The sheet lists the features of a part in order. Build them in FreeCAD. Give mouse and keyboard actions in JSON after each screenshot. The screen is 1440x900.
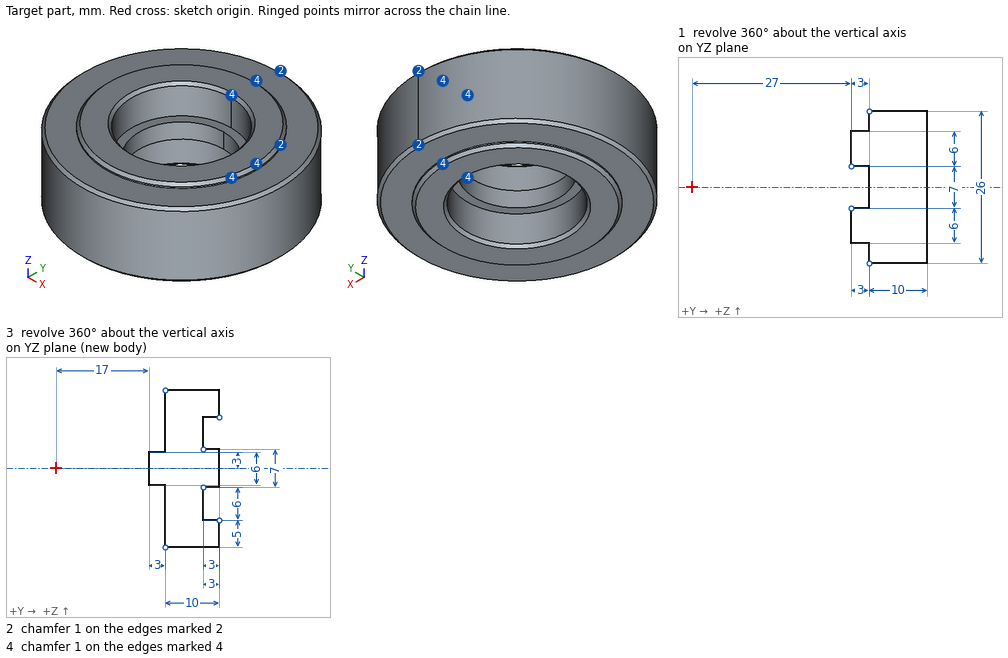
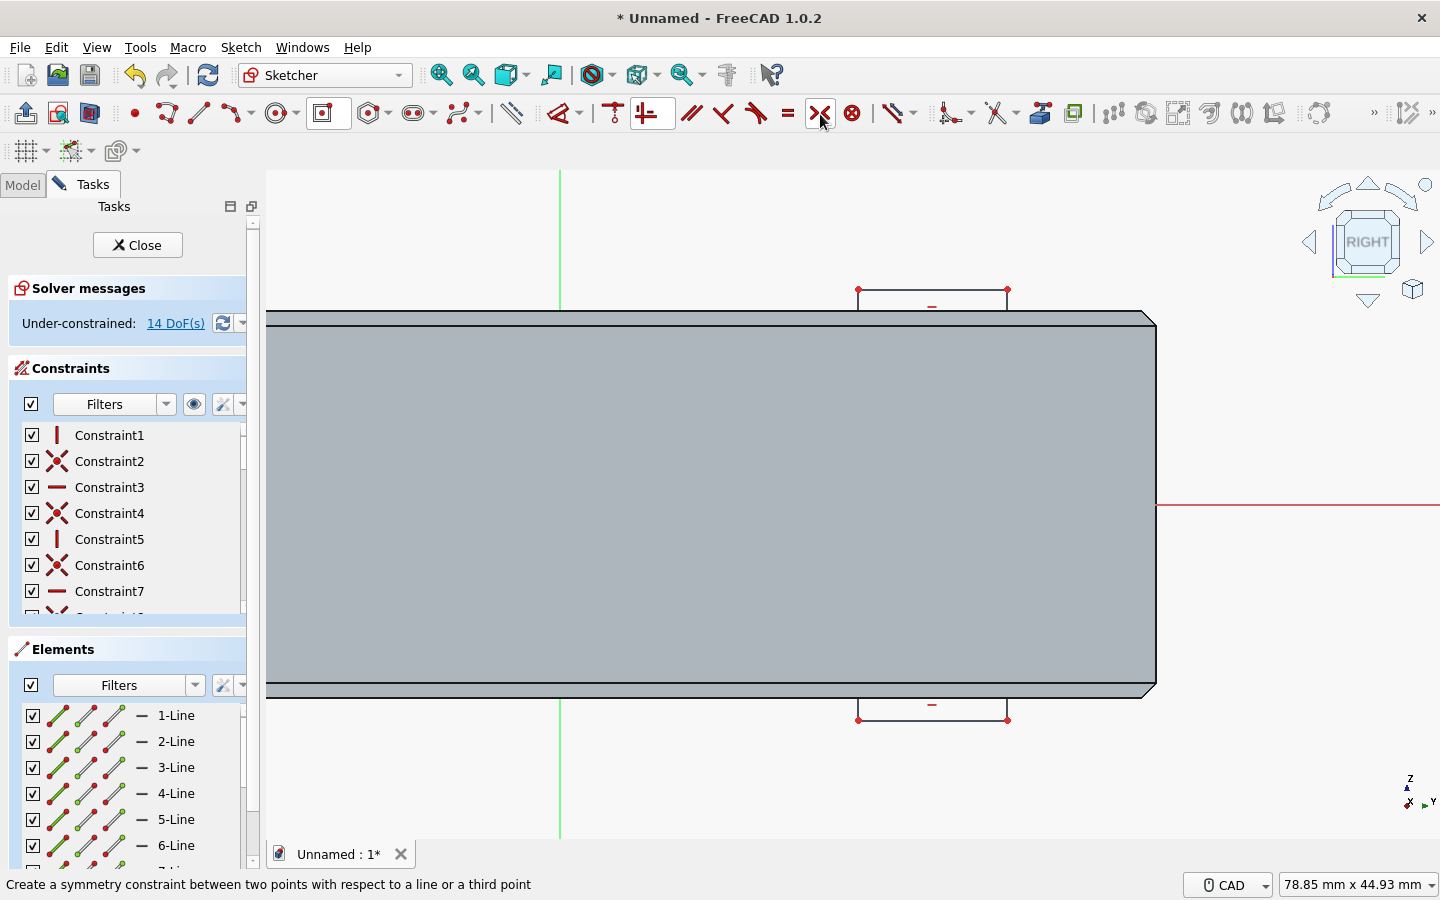
{"action": "left_click", "coordinate": [1007, 647]}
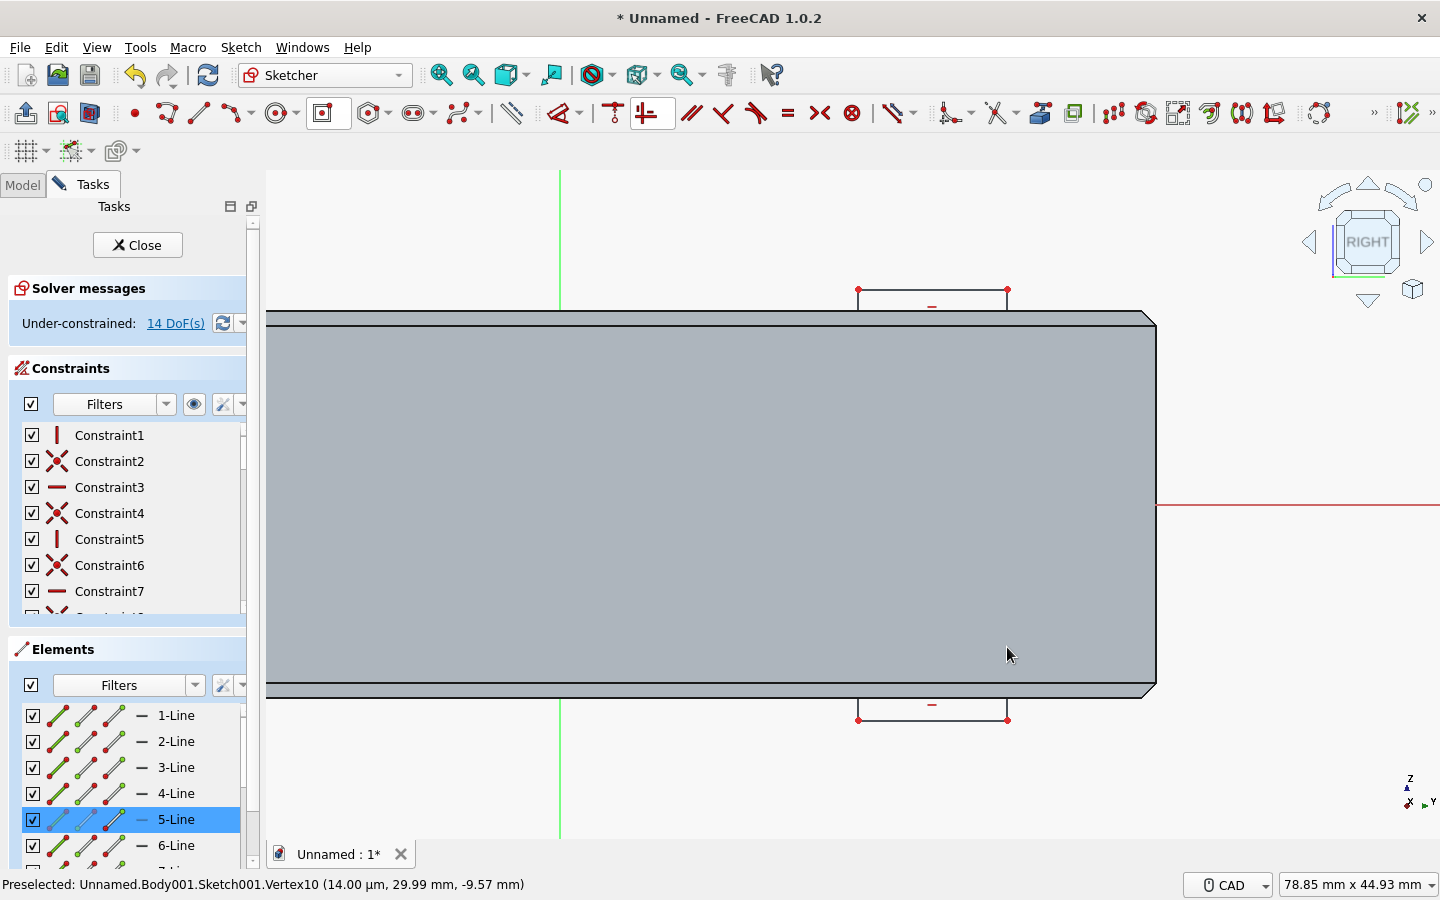
{"action": "left_click", "coordinate": [1007, 364]}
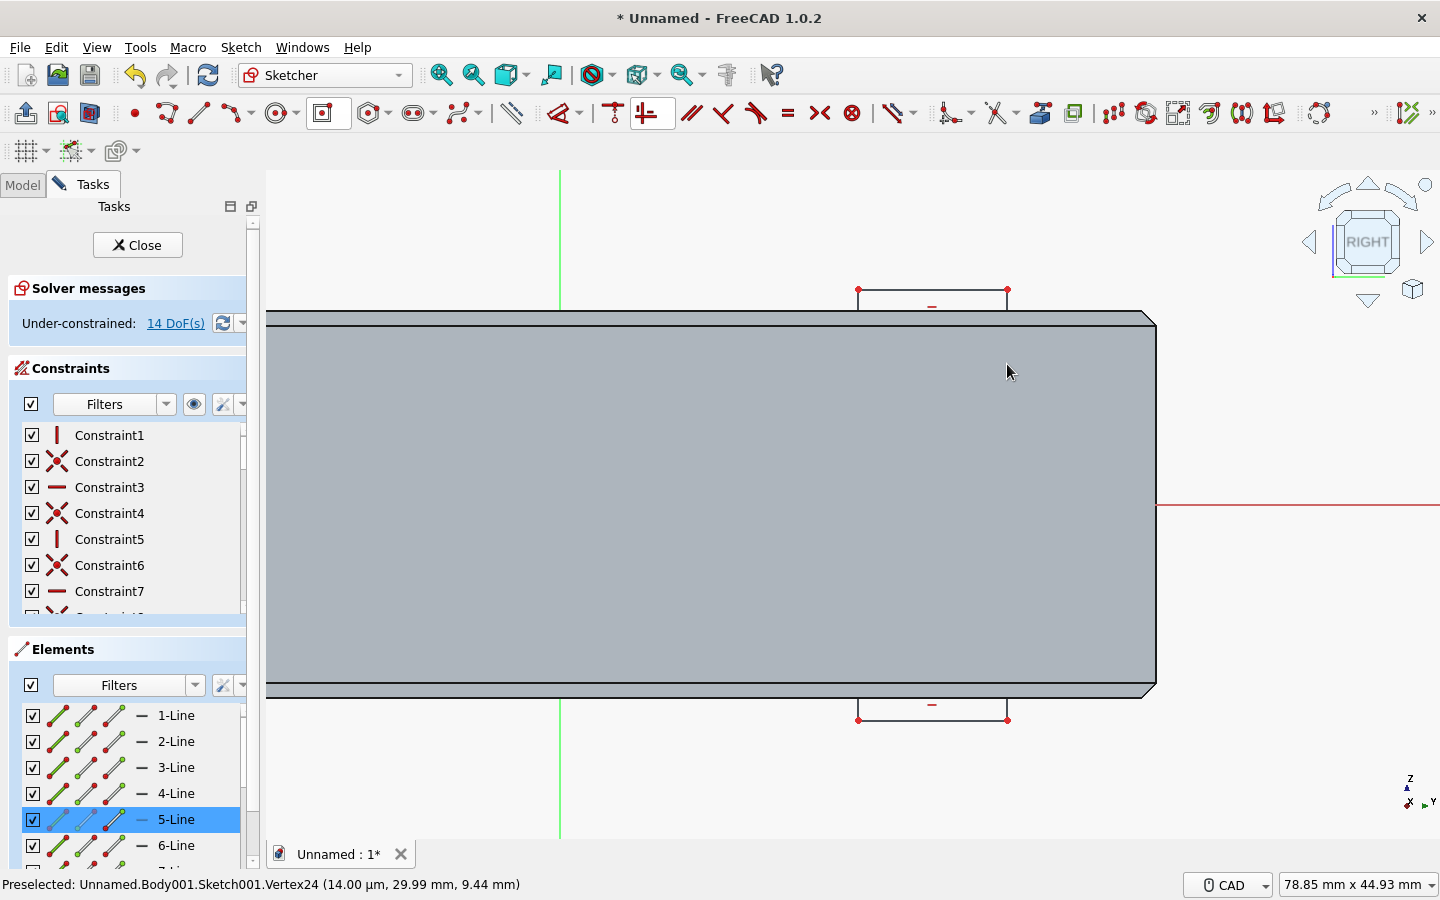
{"action": "left_click", "coordinate": [364, 504]}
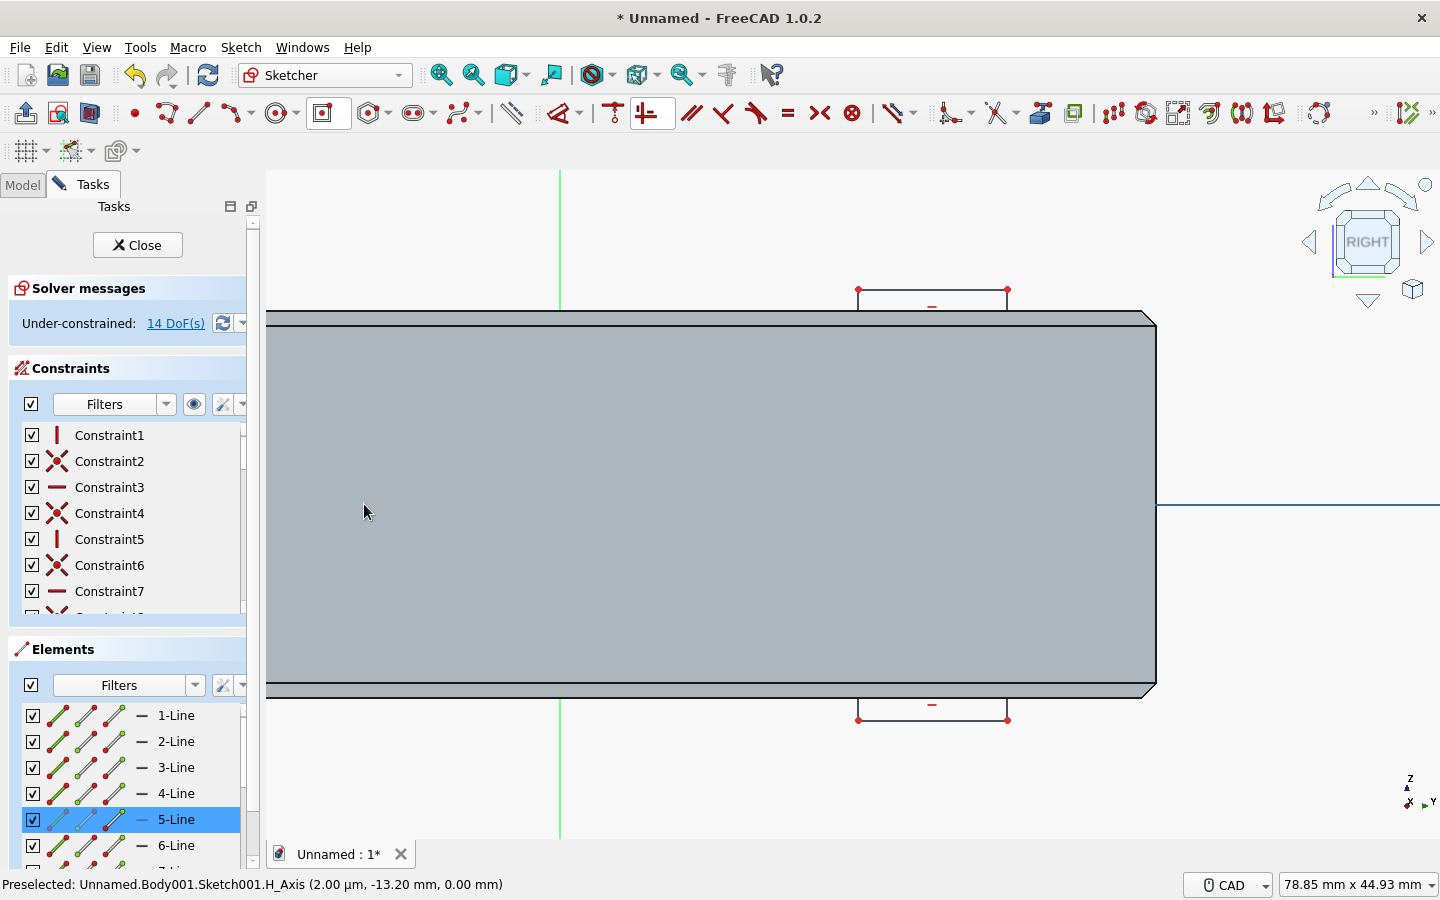
{"action": "left_click", "coordinate": [820, 114]}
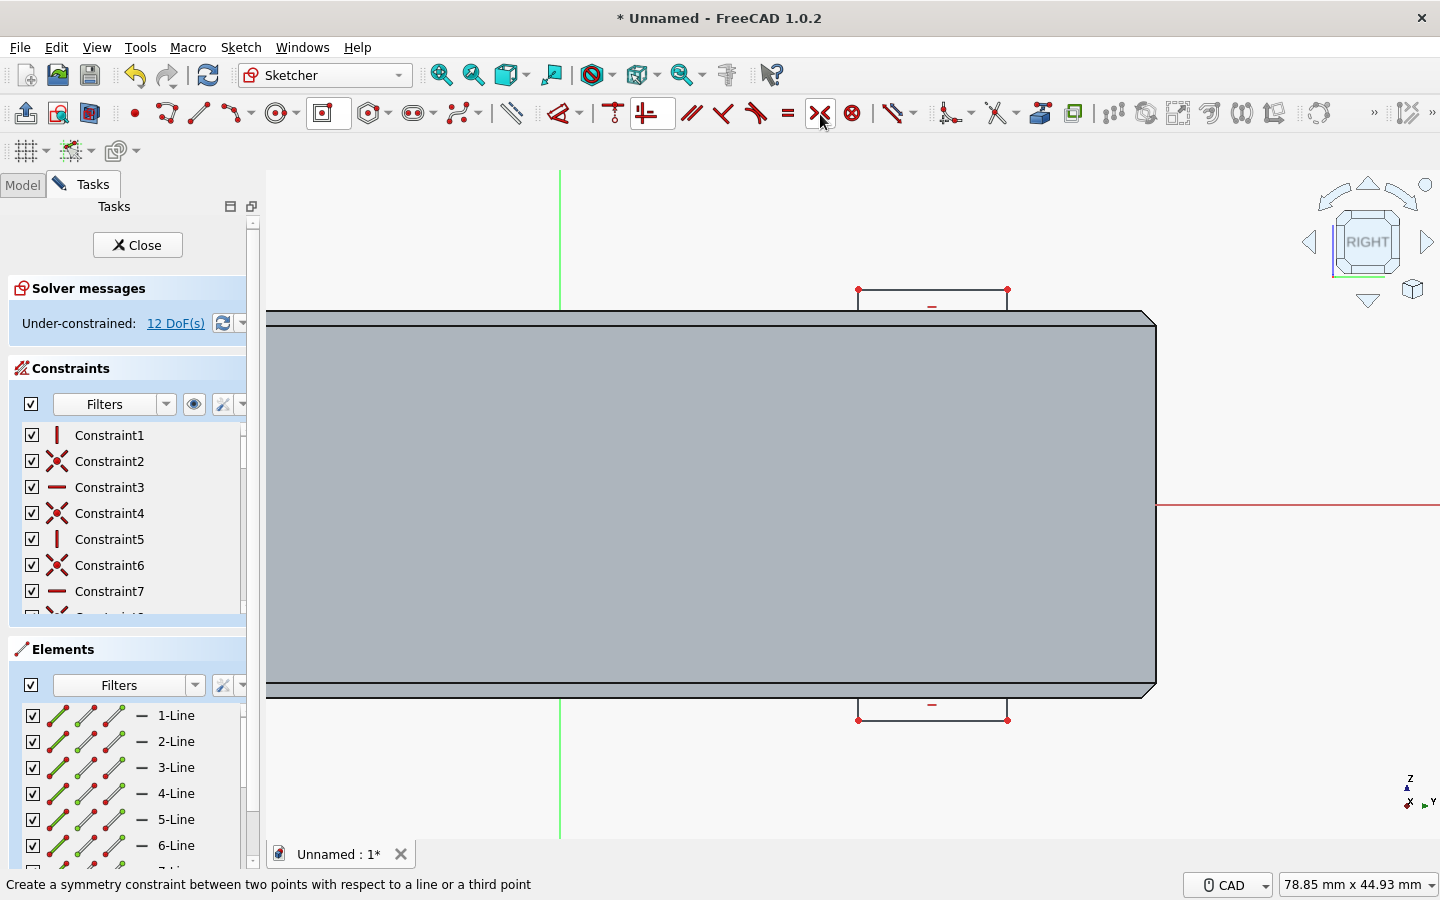
{"action": "left_click", "coordinate": [858, 721]}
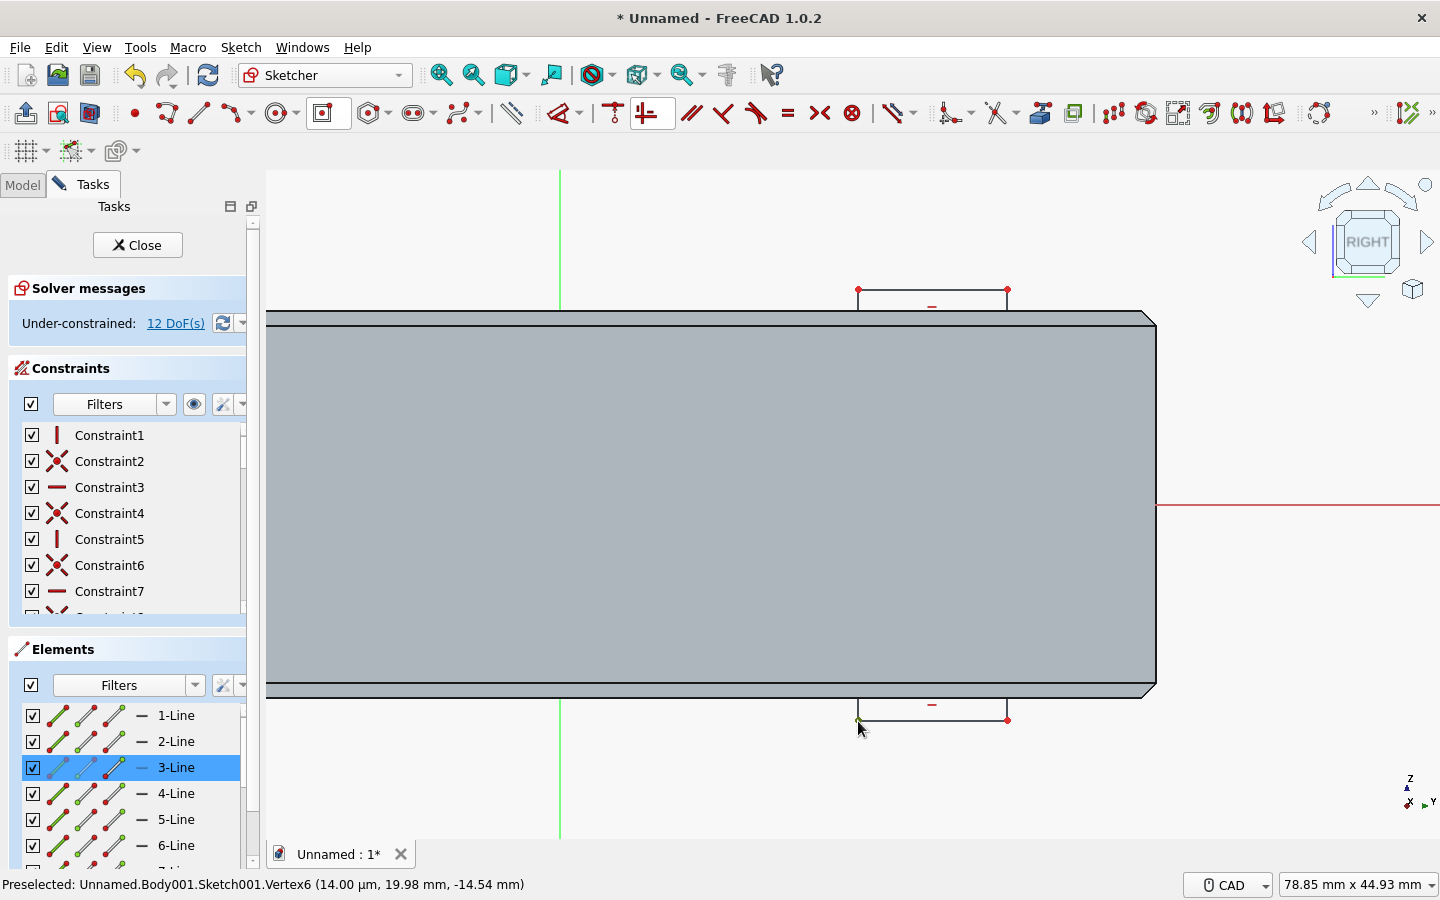
{"action": "left_click", "coordinate": [858, 290]}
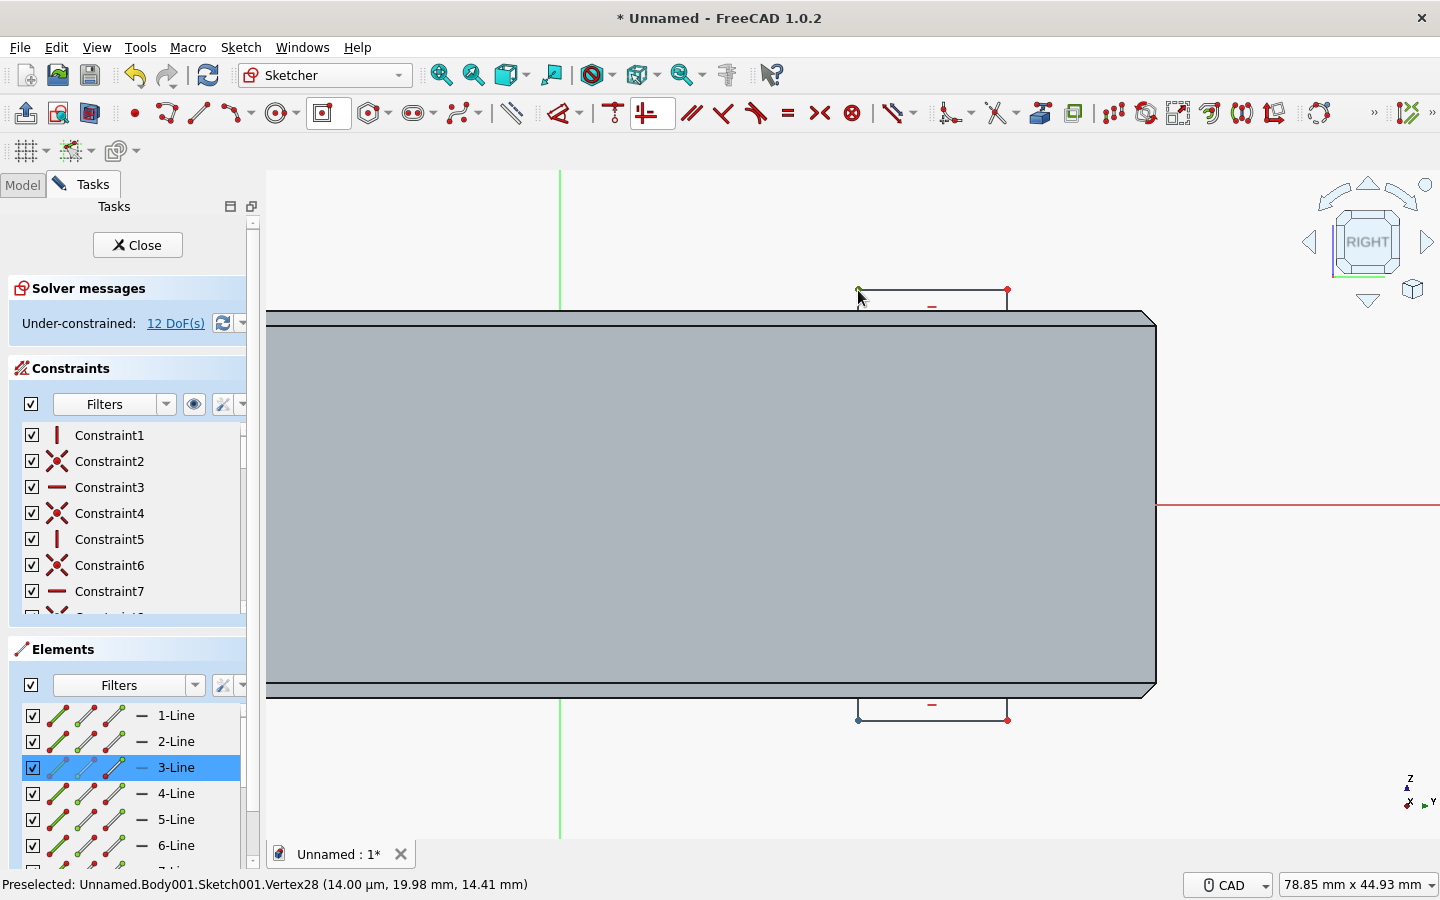
{"action": "left_click", "coordinate": [364, 504]}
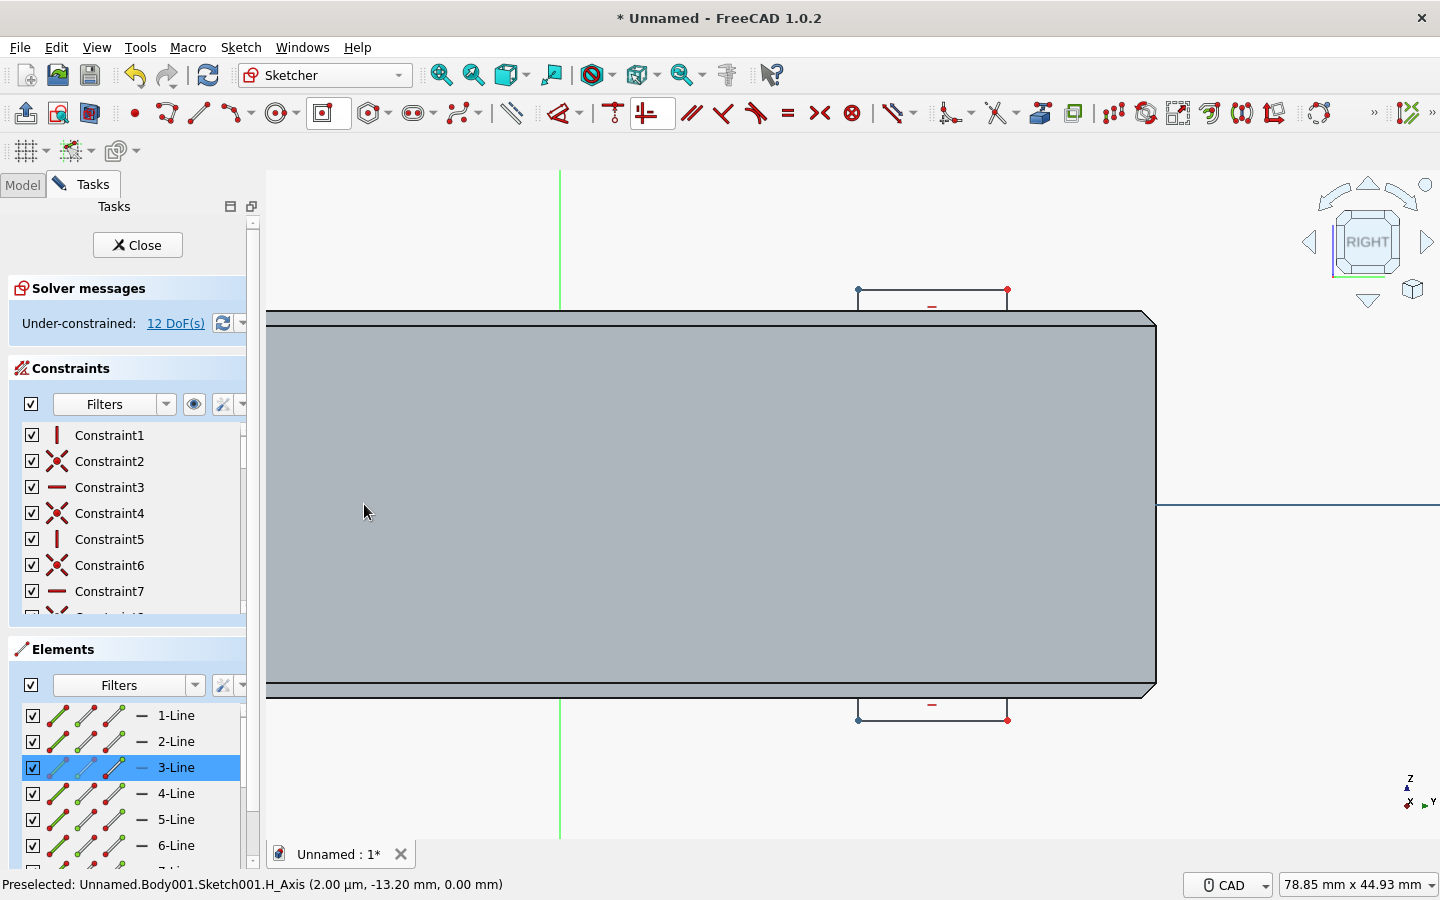
{"action": "left_click", "coordinate": [820, 114]}